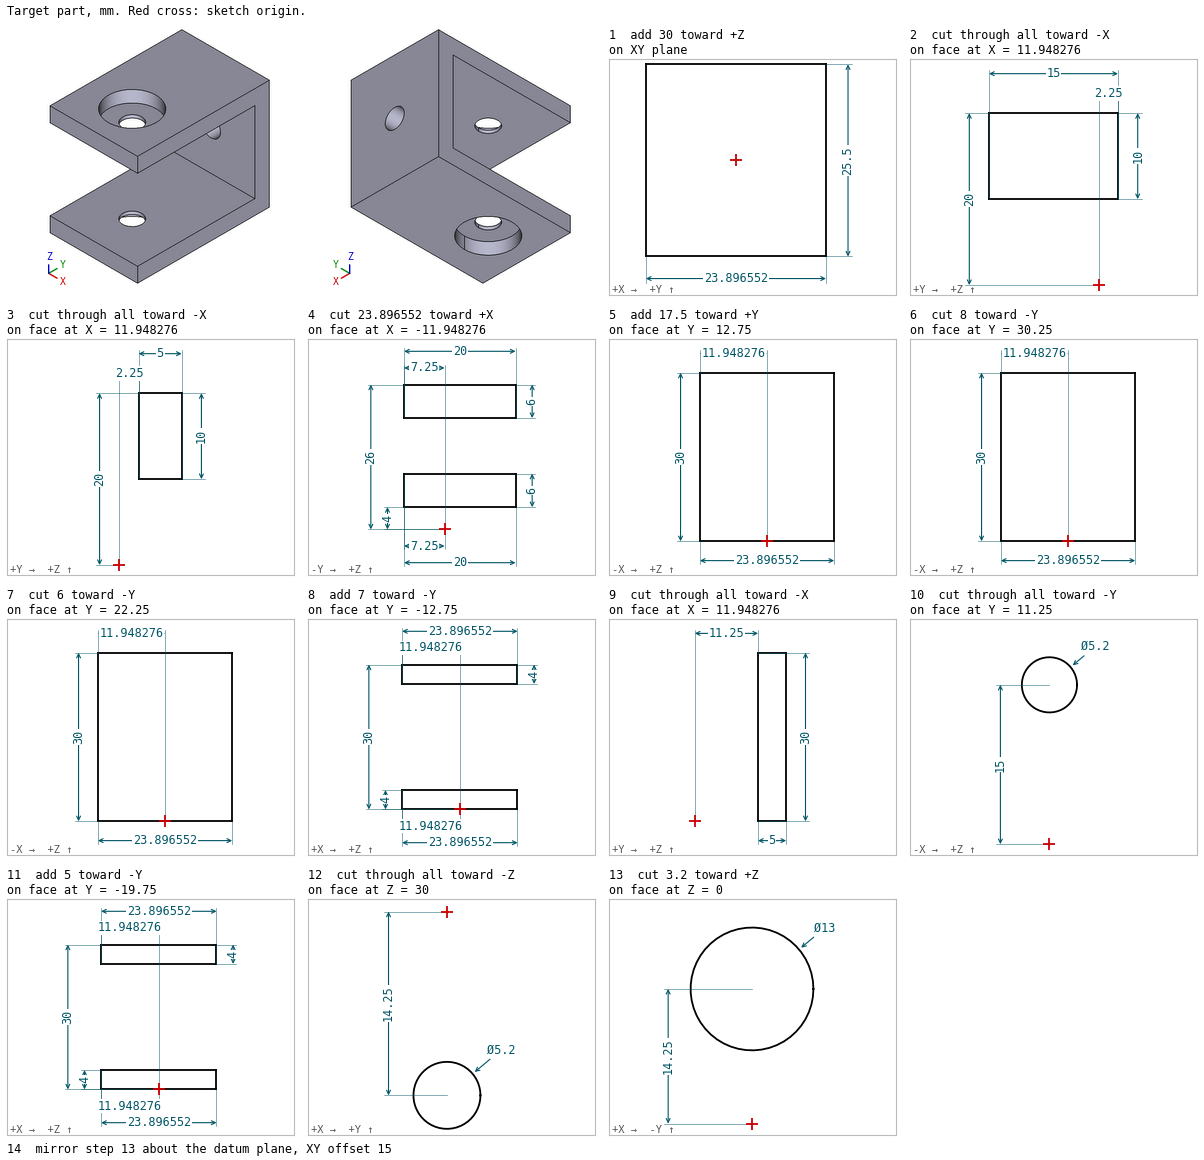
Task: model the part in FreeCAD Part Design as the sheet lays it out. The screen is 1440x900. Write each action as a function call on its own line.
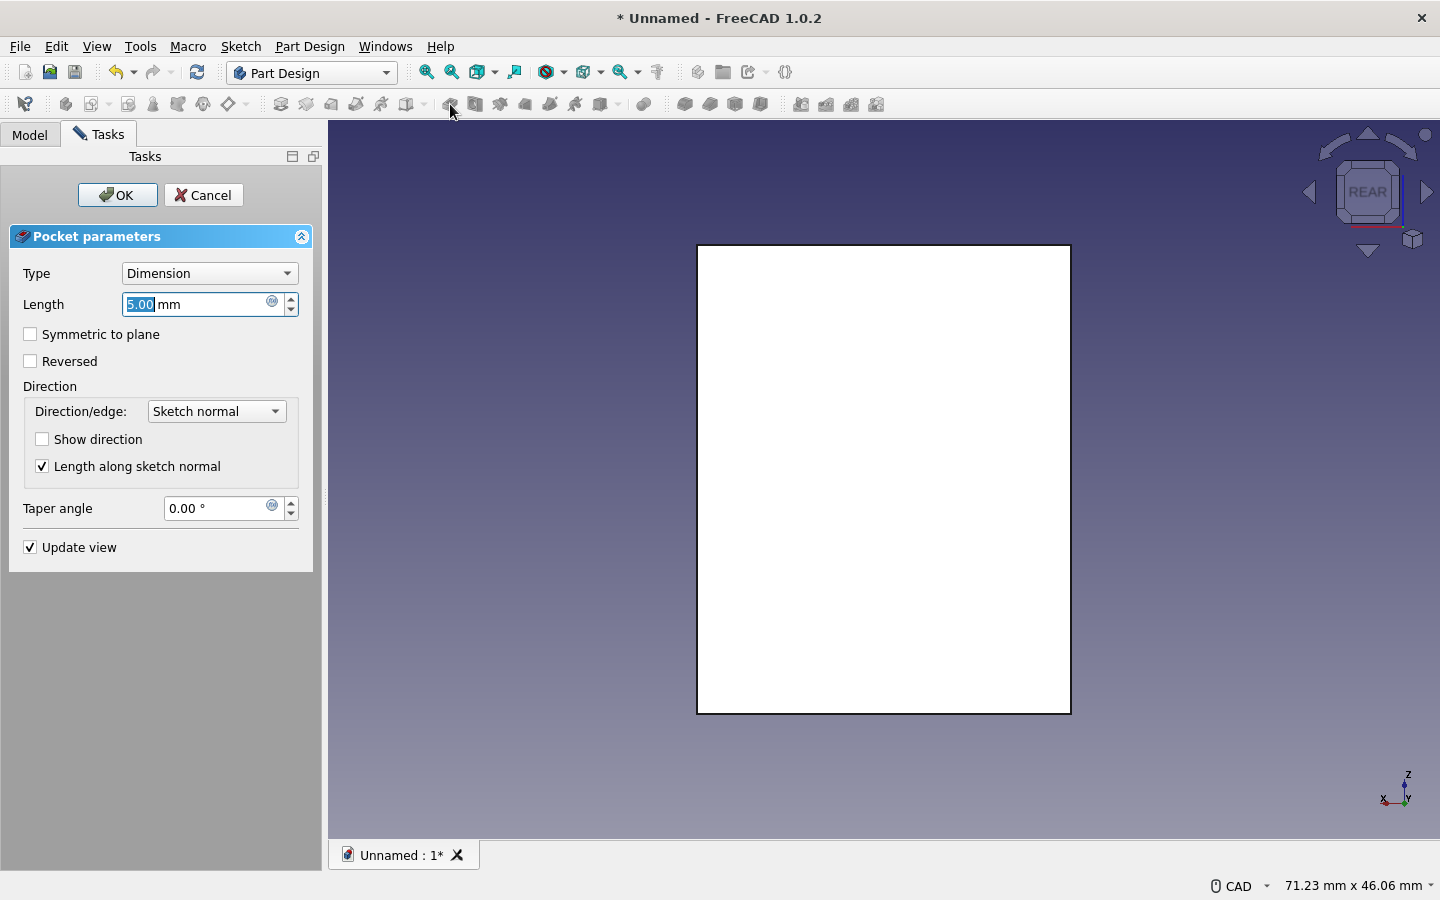
text(6)
key(Tab)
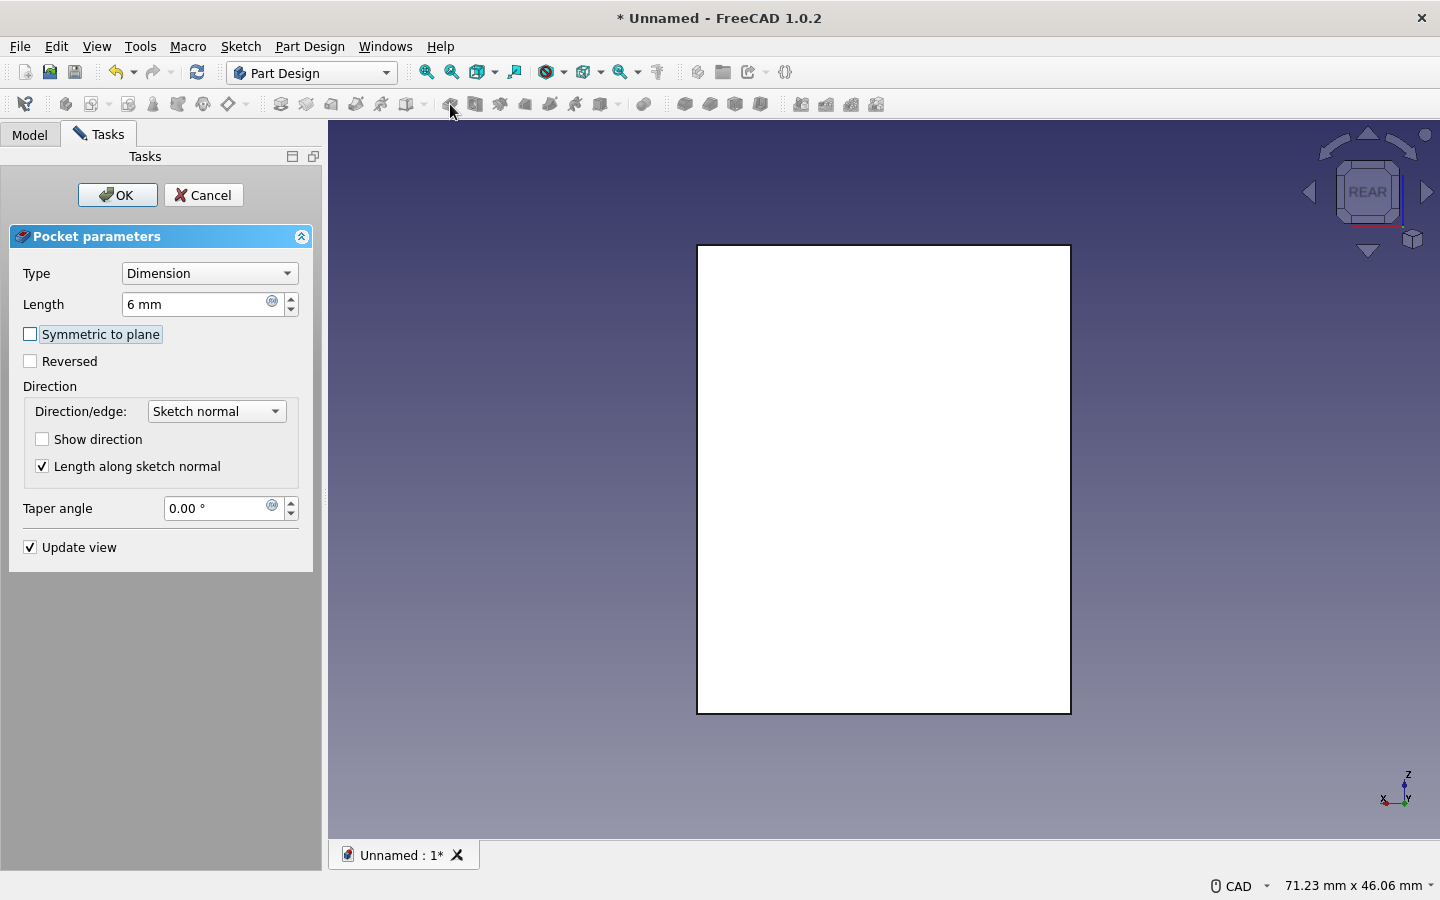
click(118, 195)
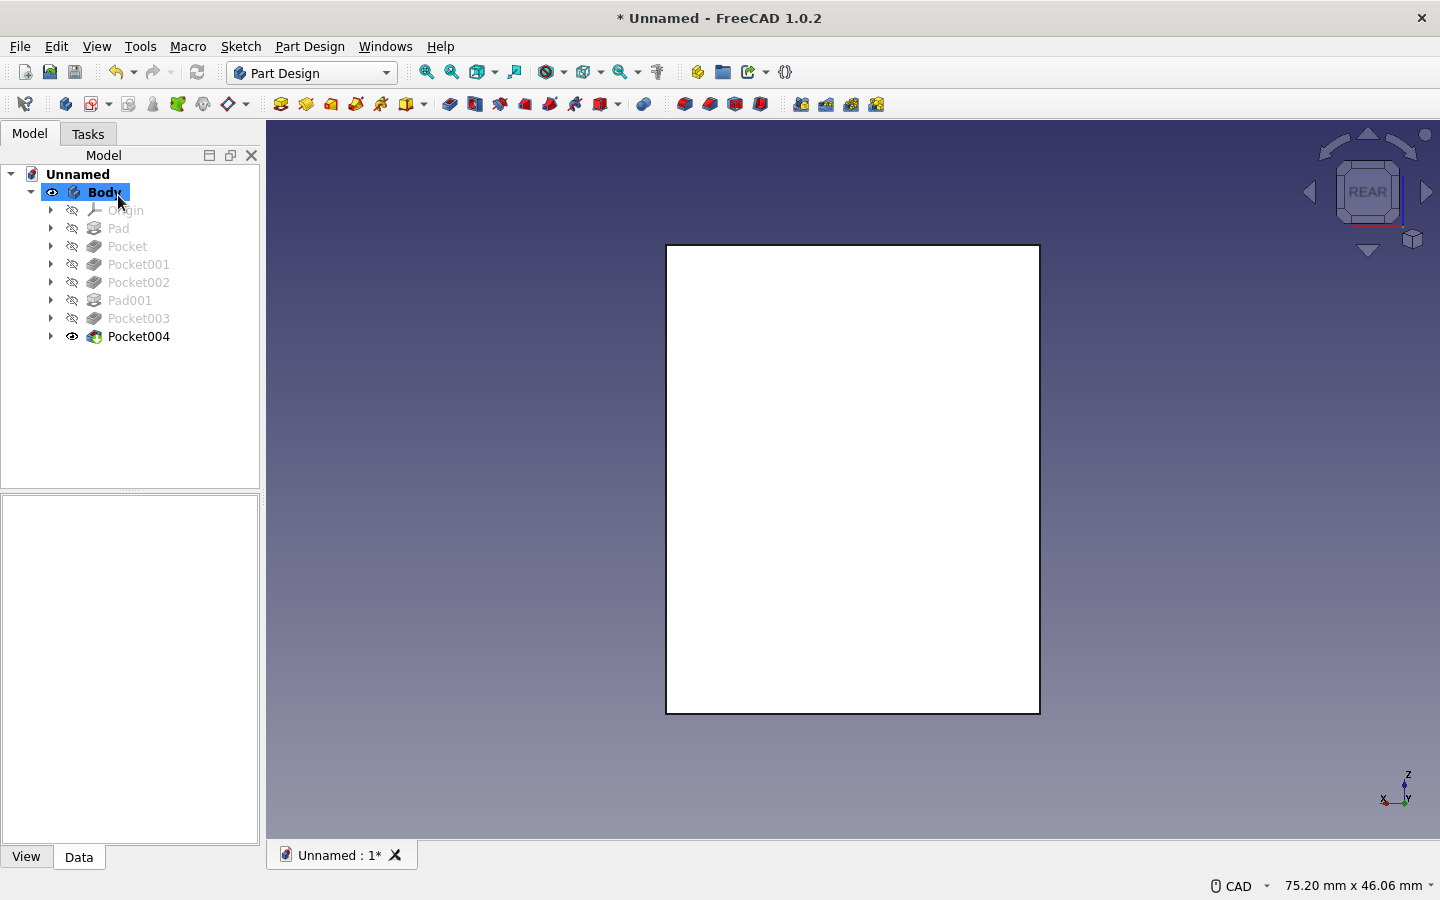
key(0)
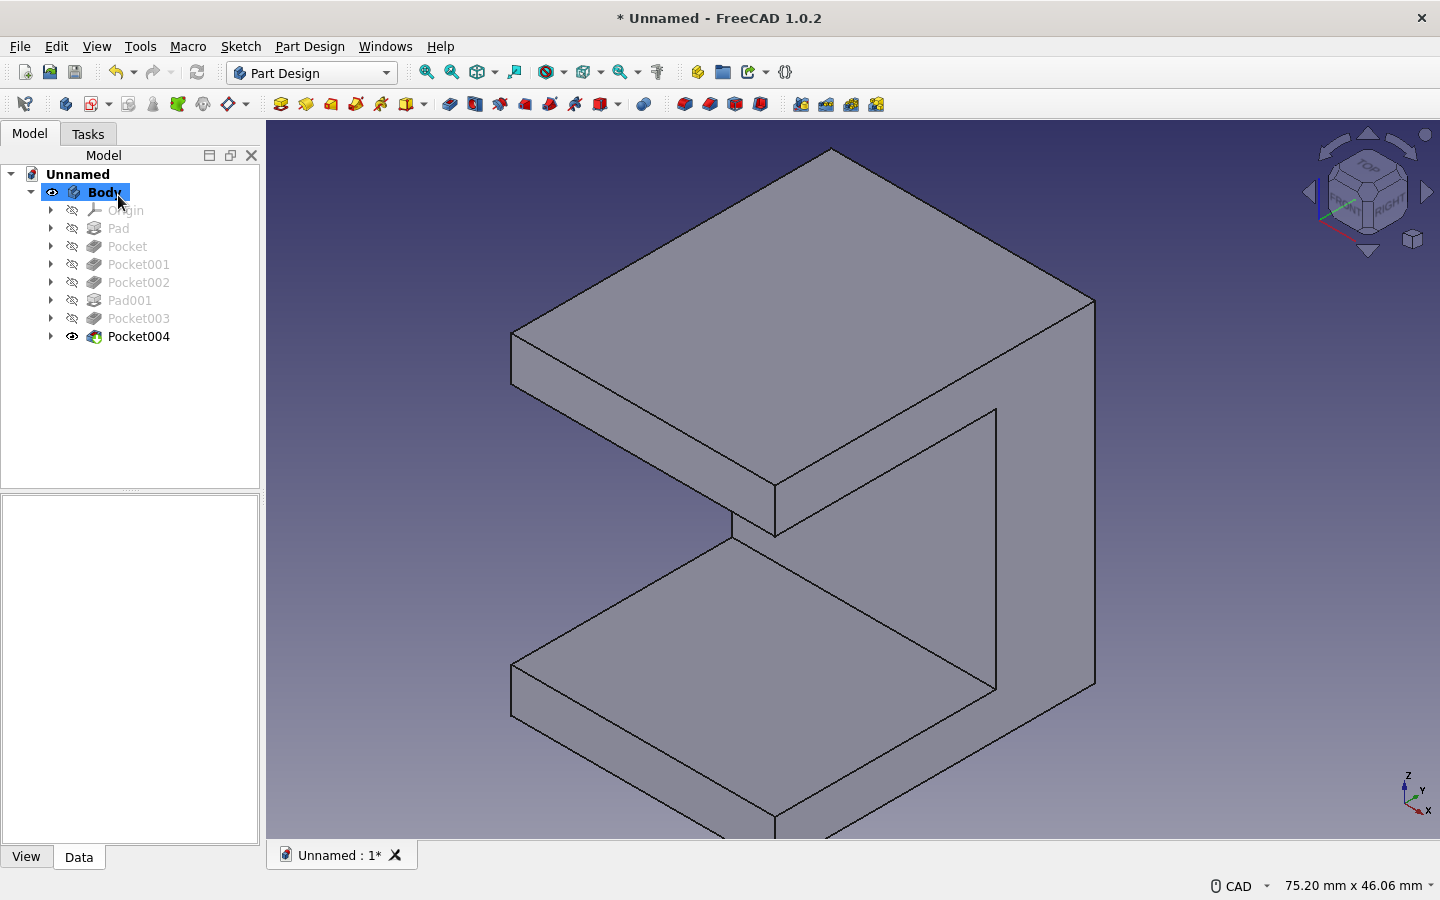
key(v)
key(f)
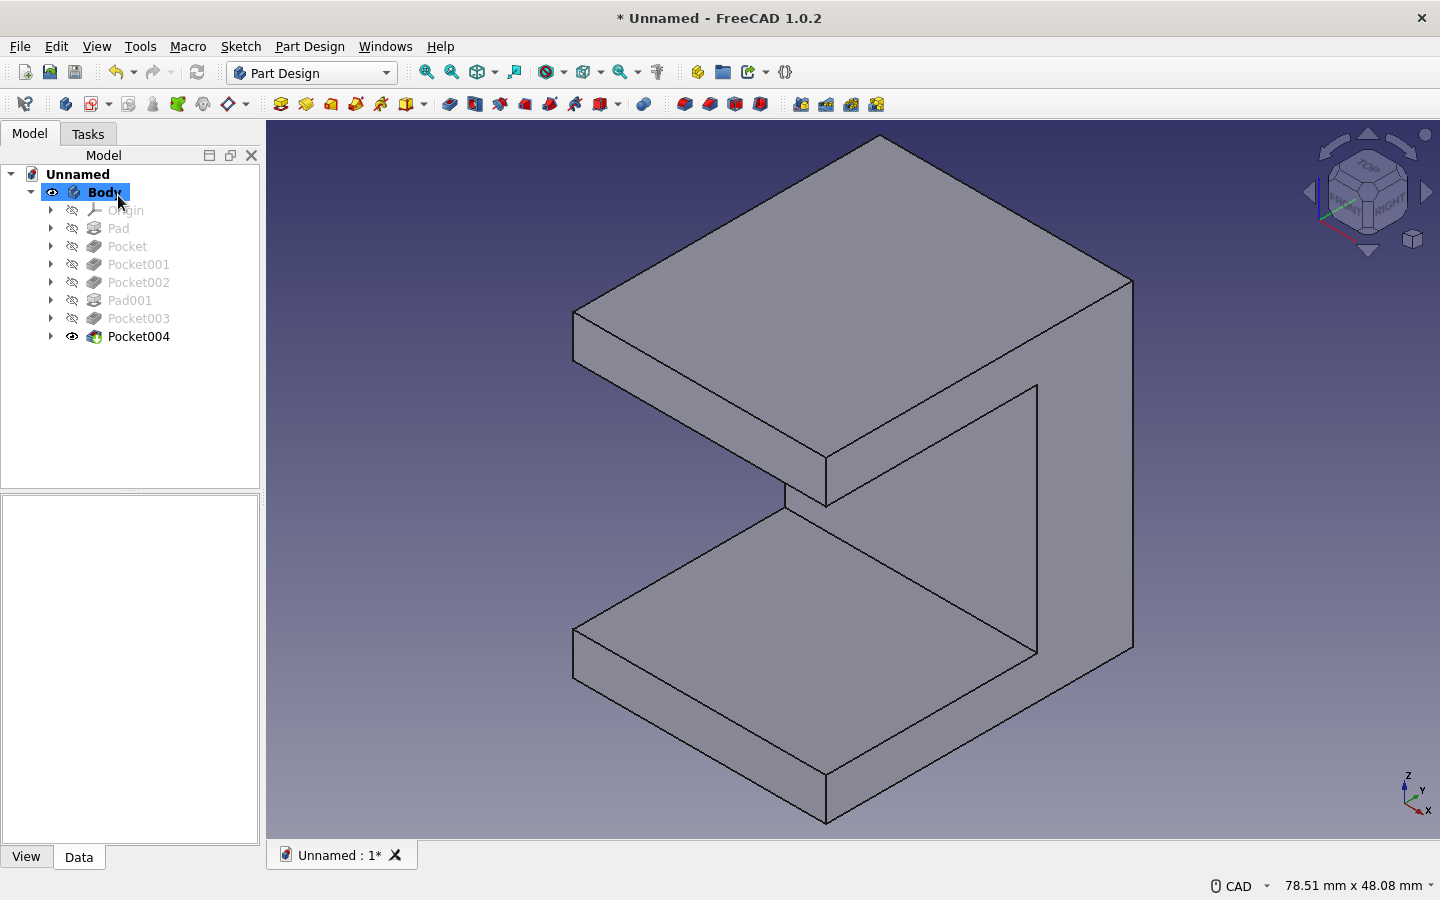
click(772, 767)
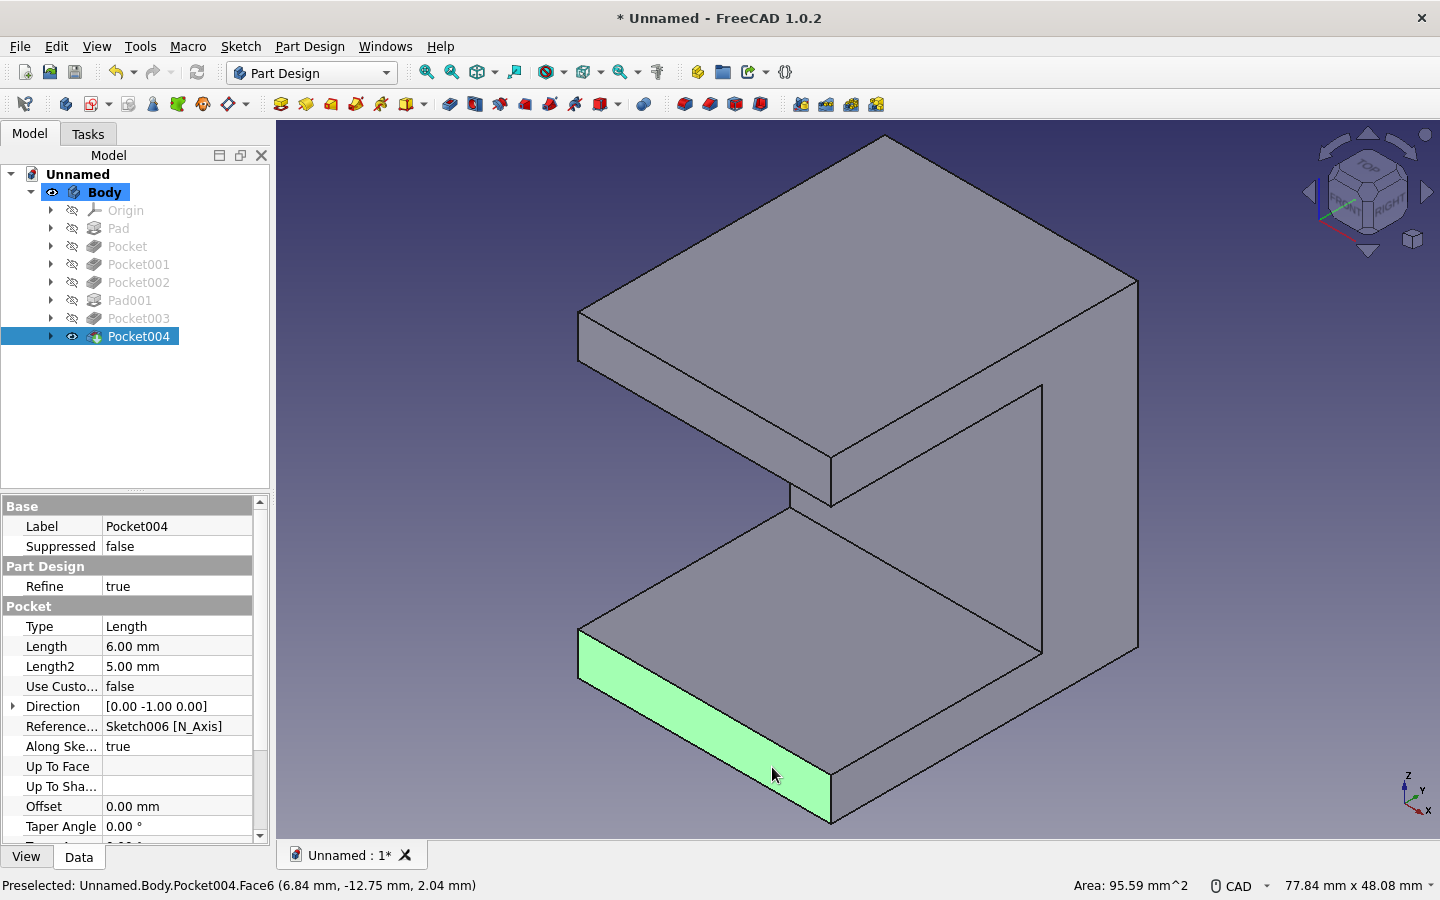
click(90, 104)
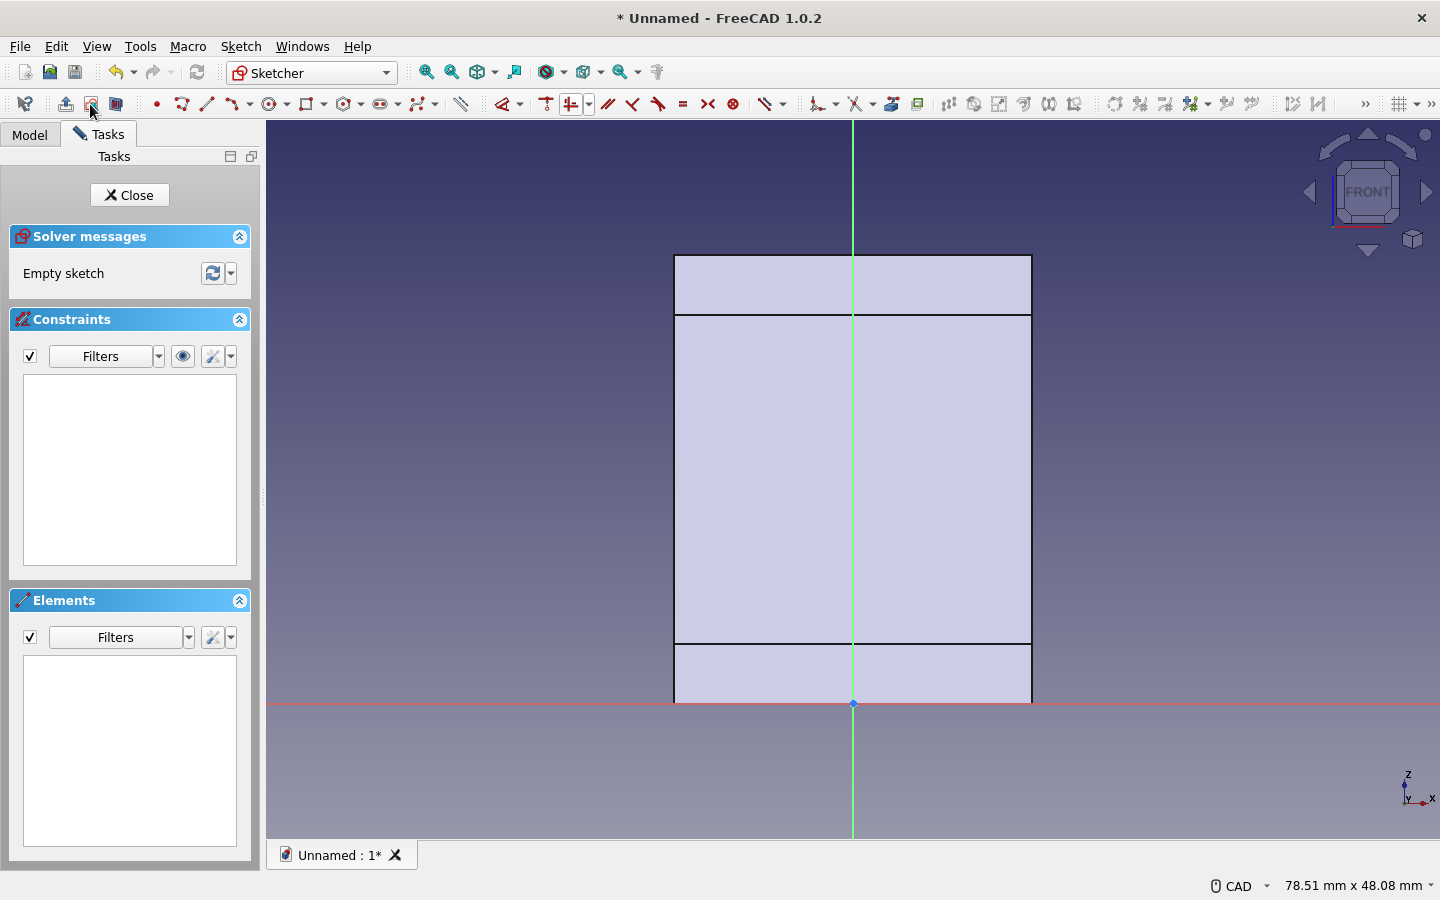
click(306, 104)